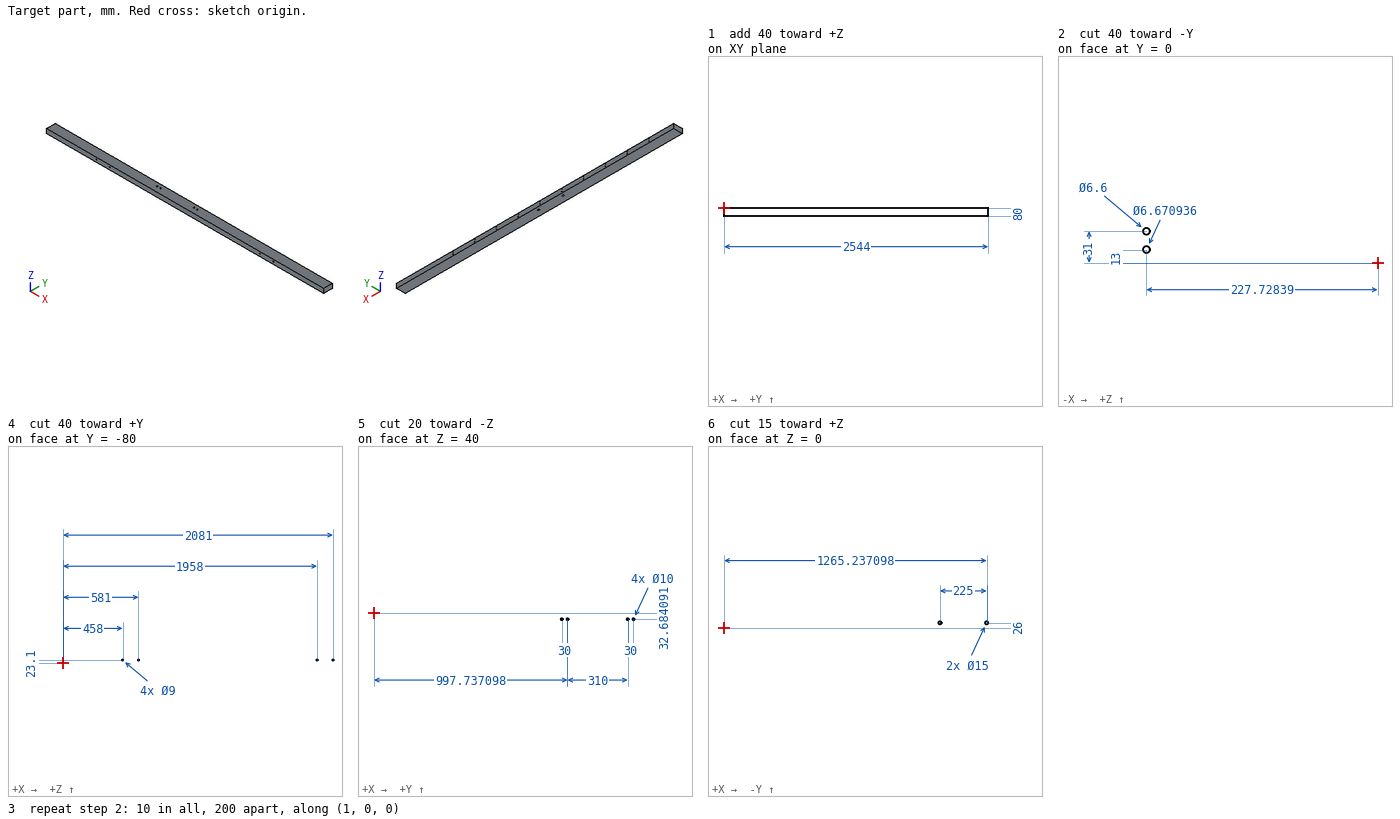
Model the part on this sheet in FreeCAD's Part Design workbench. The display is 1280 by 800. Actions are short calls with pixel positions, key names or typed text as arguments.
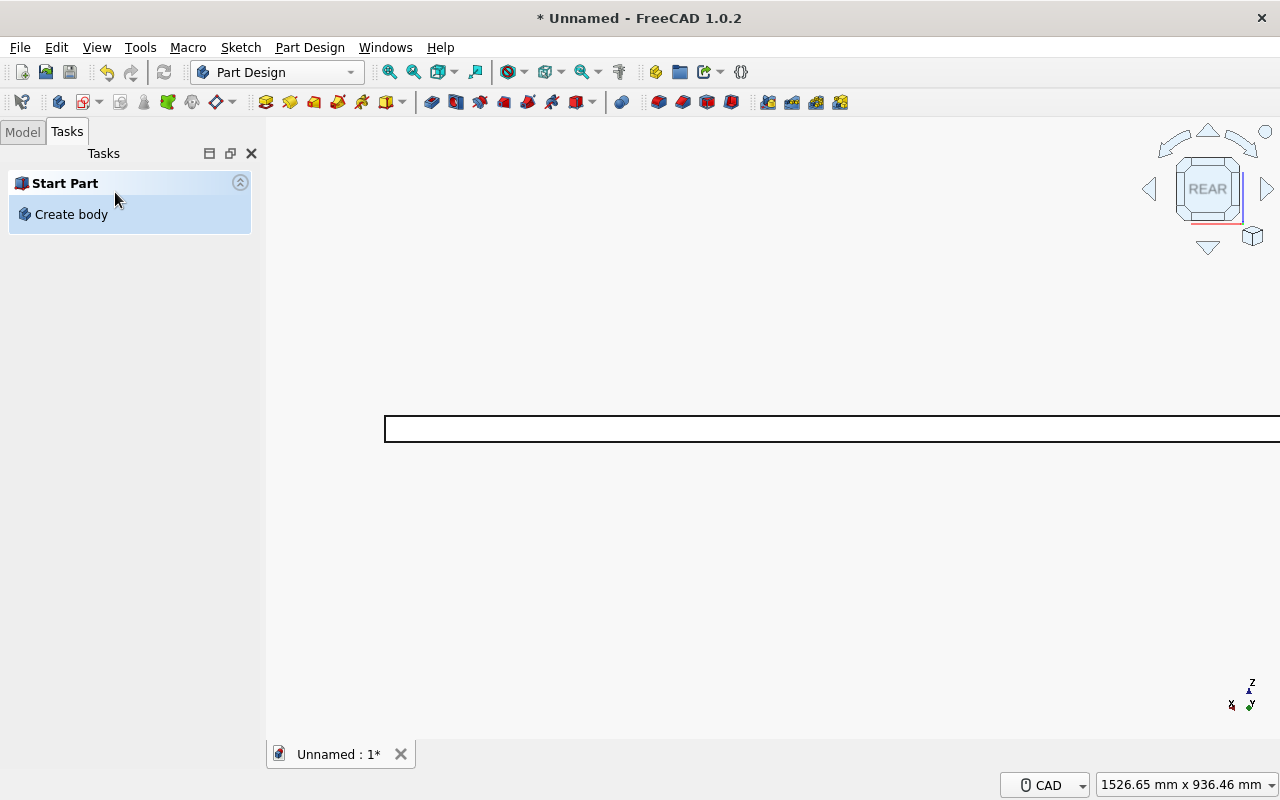
key(v)
key(f)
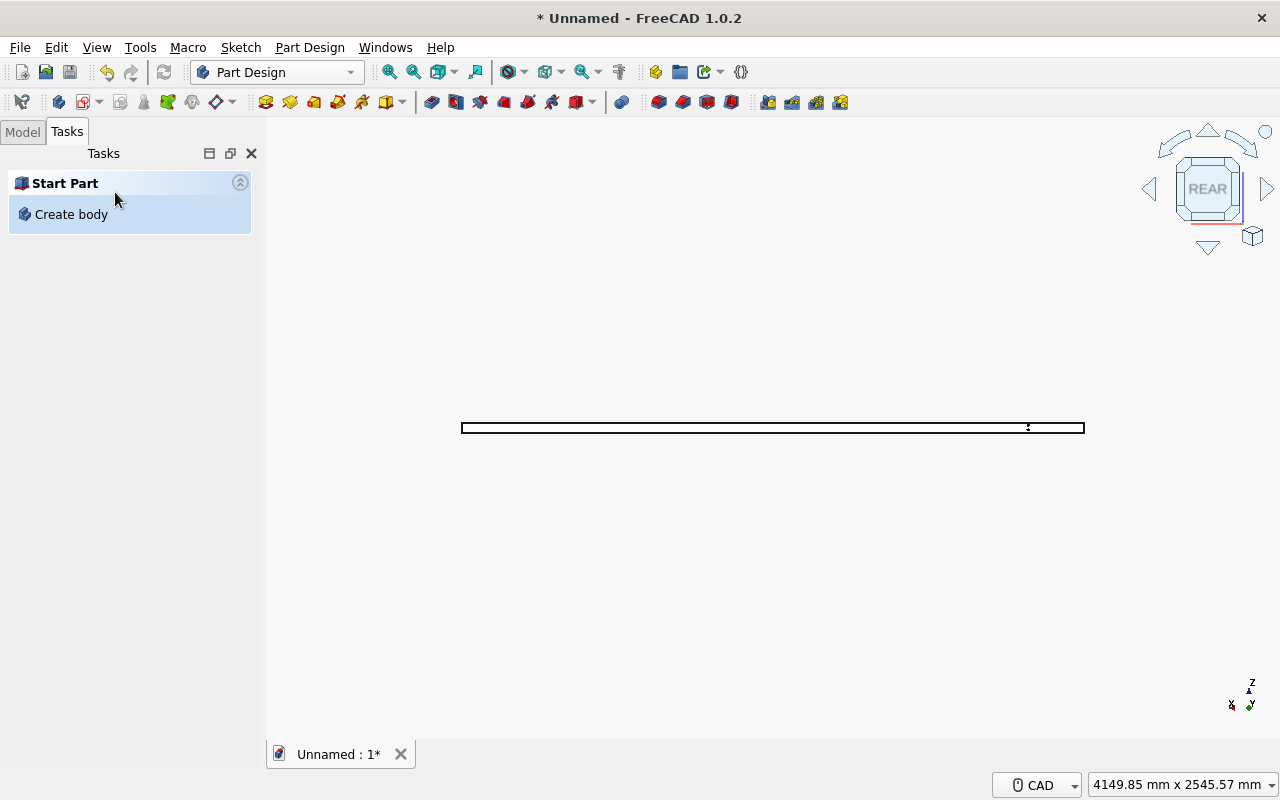
click(23, 131)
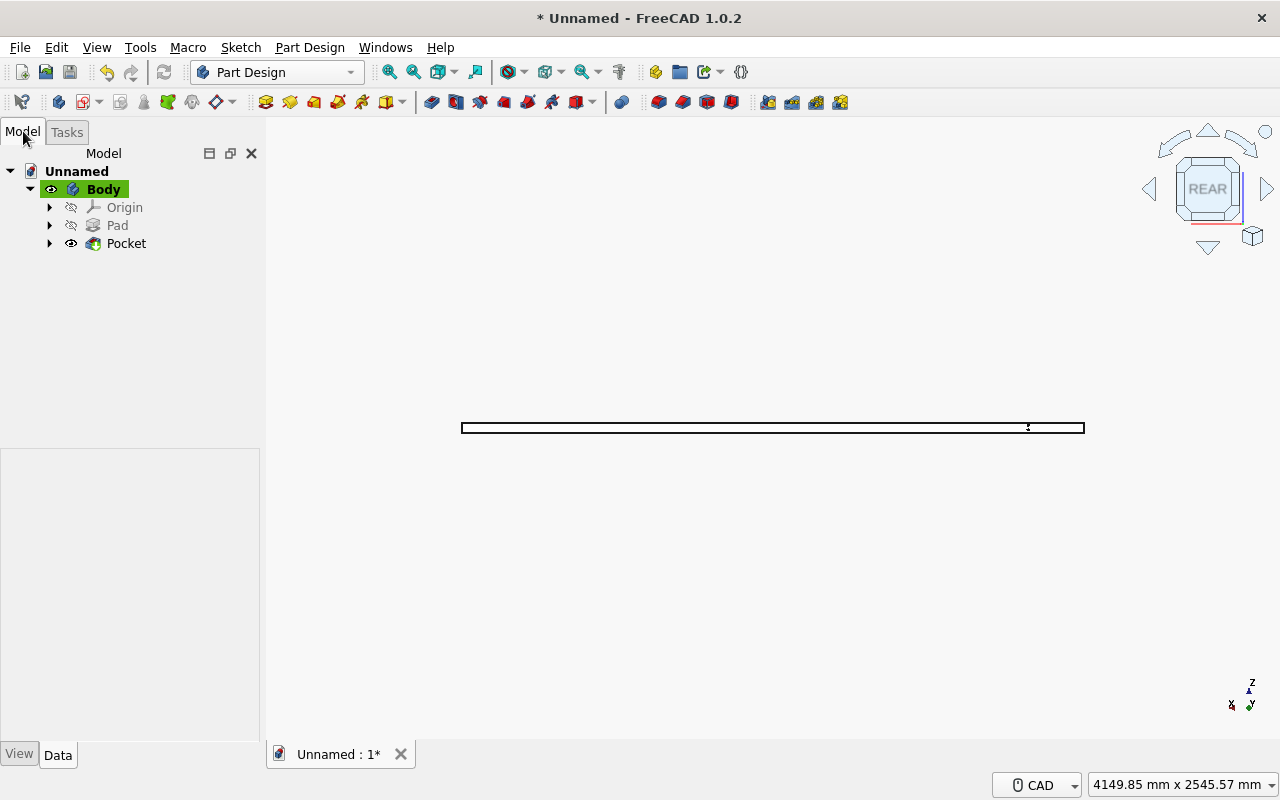
click(116, 243)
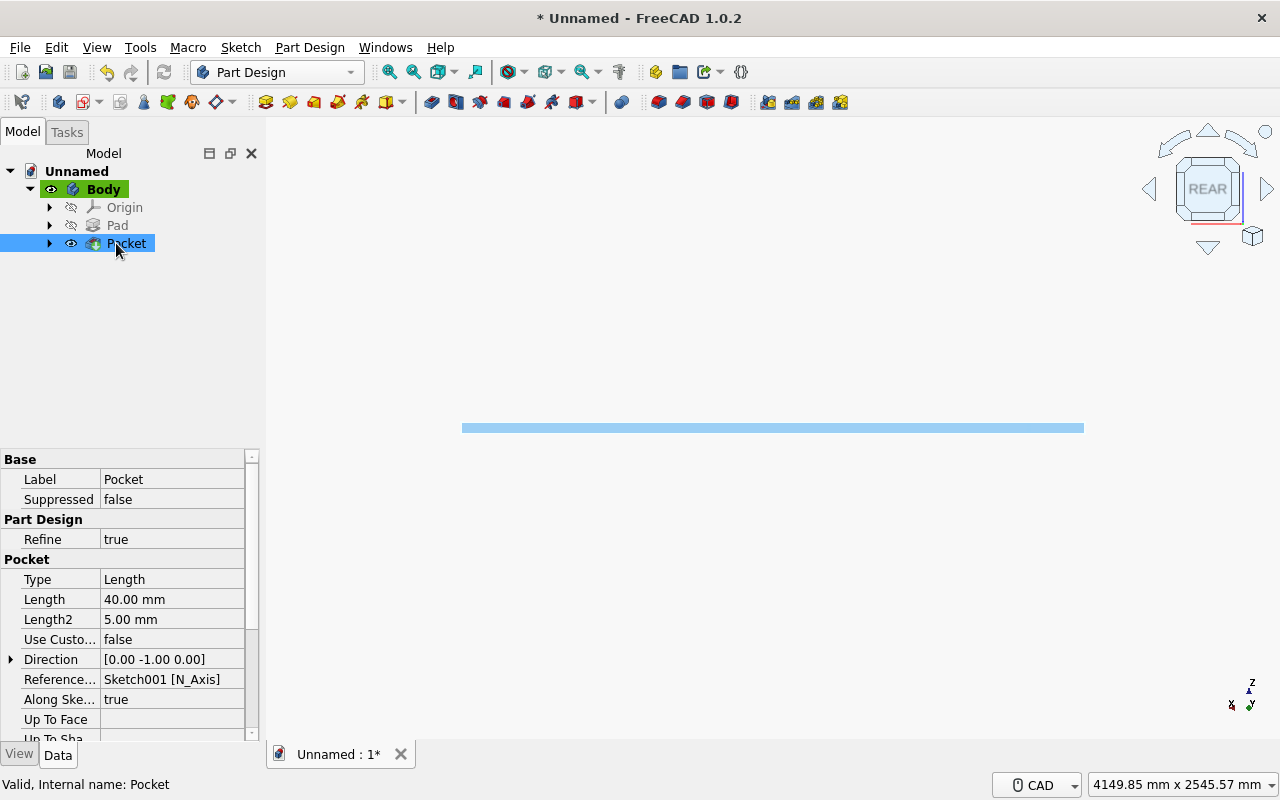
click(792, 102)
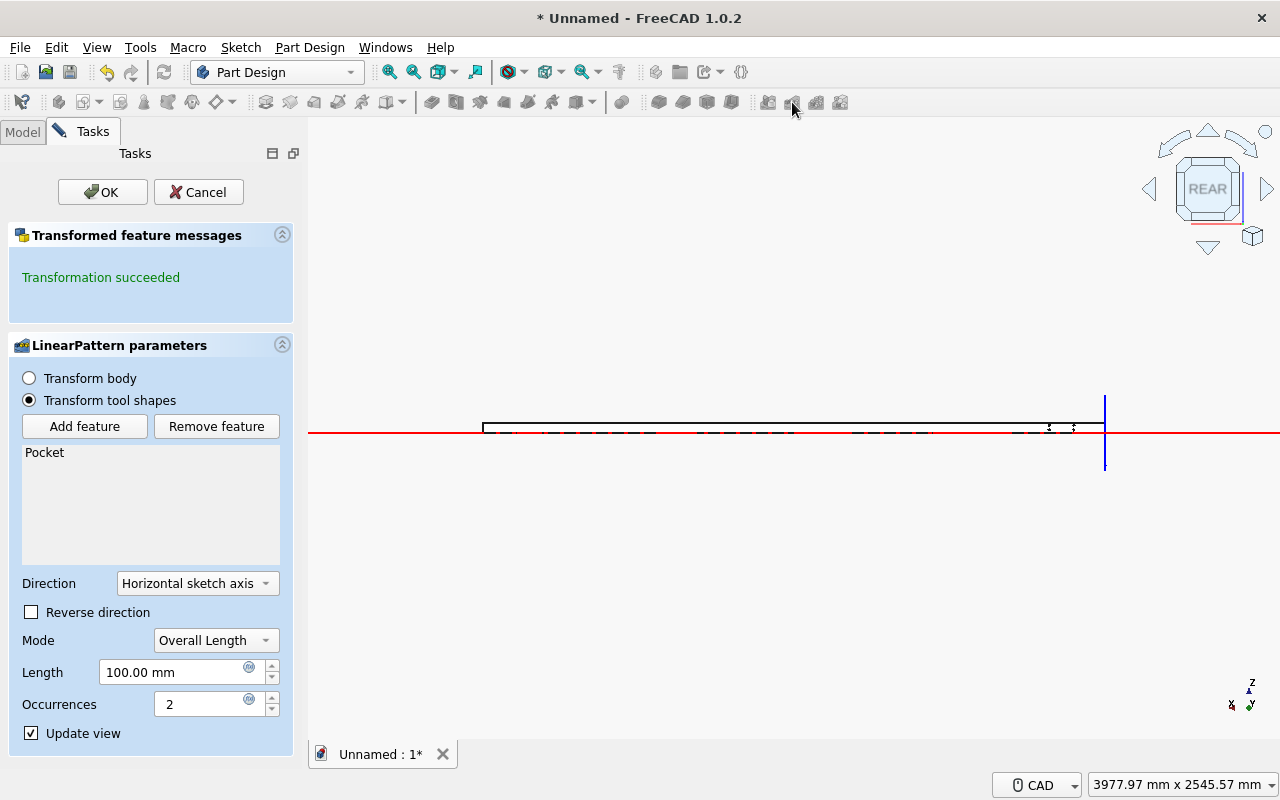
click(198, 584)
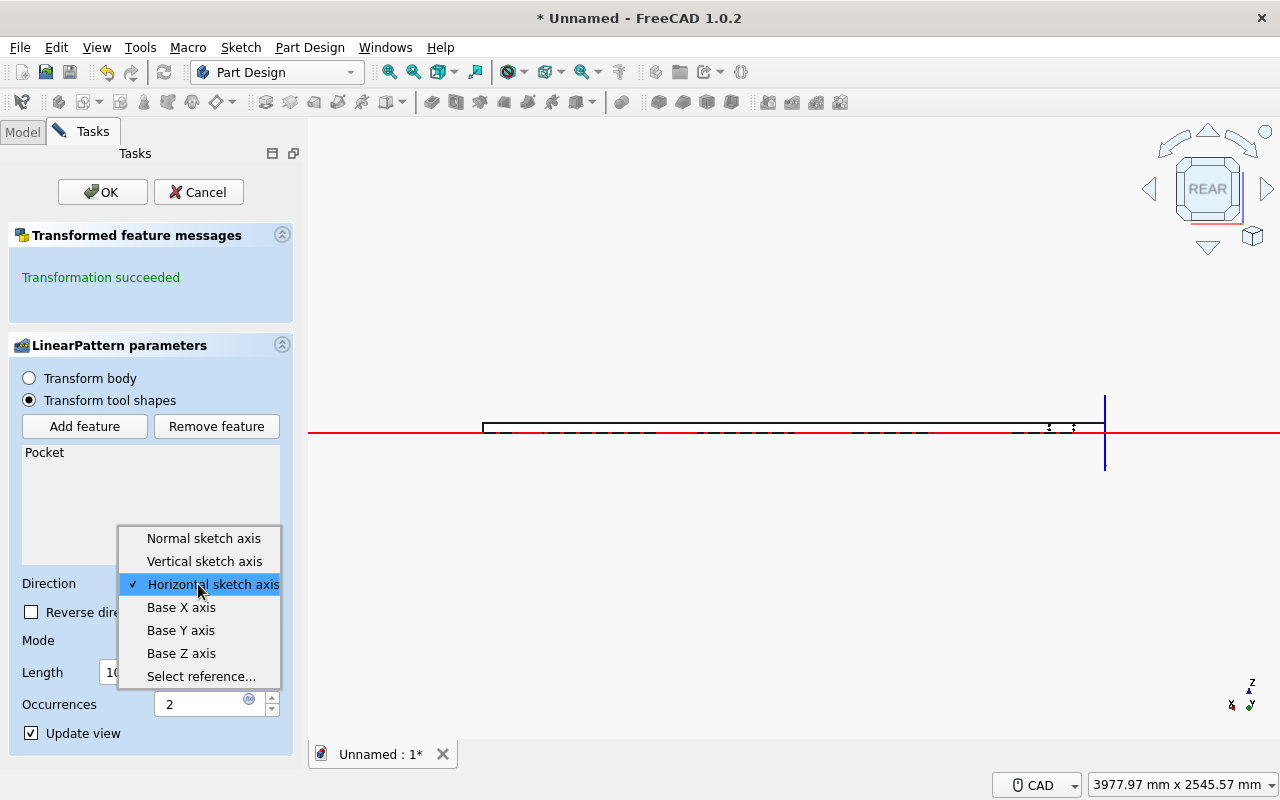
click(198, 608)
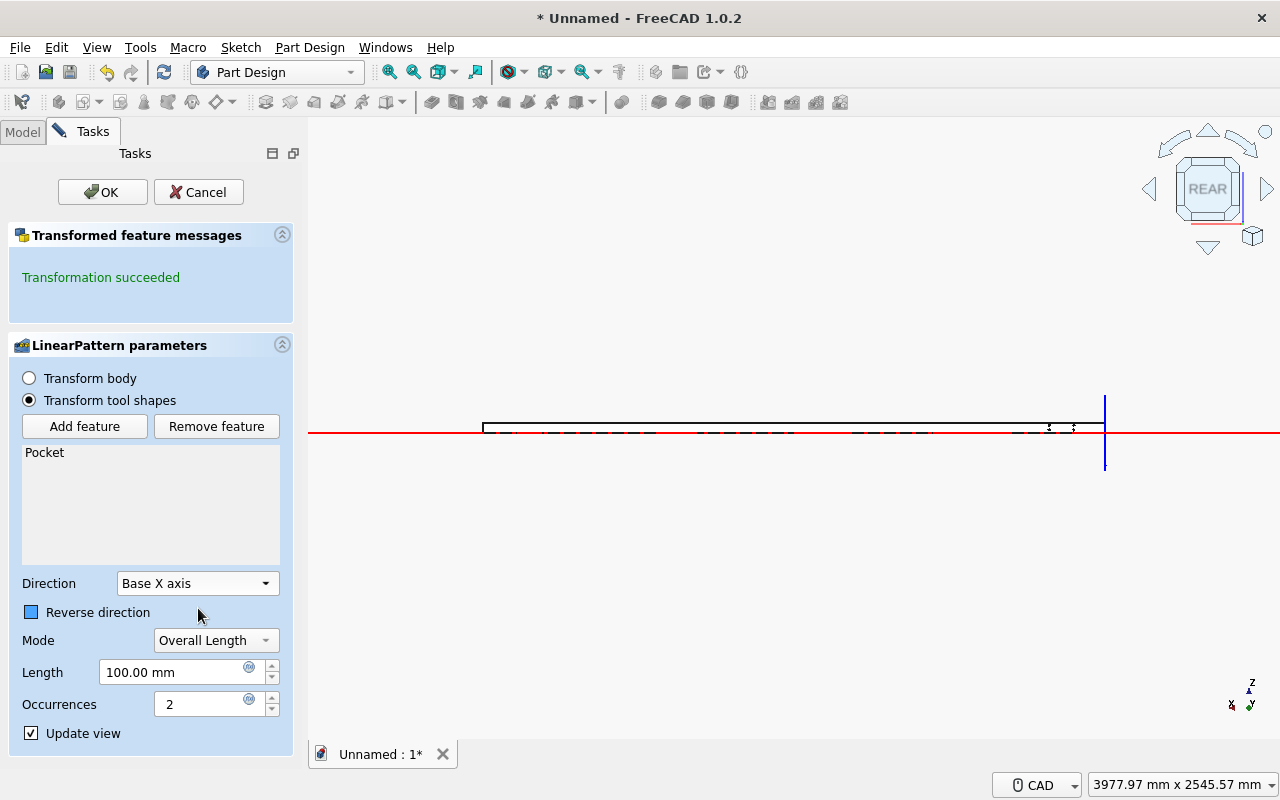
click(217, 640)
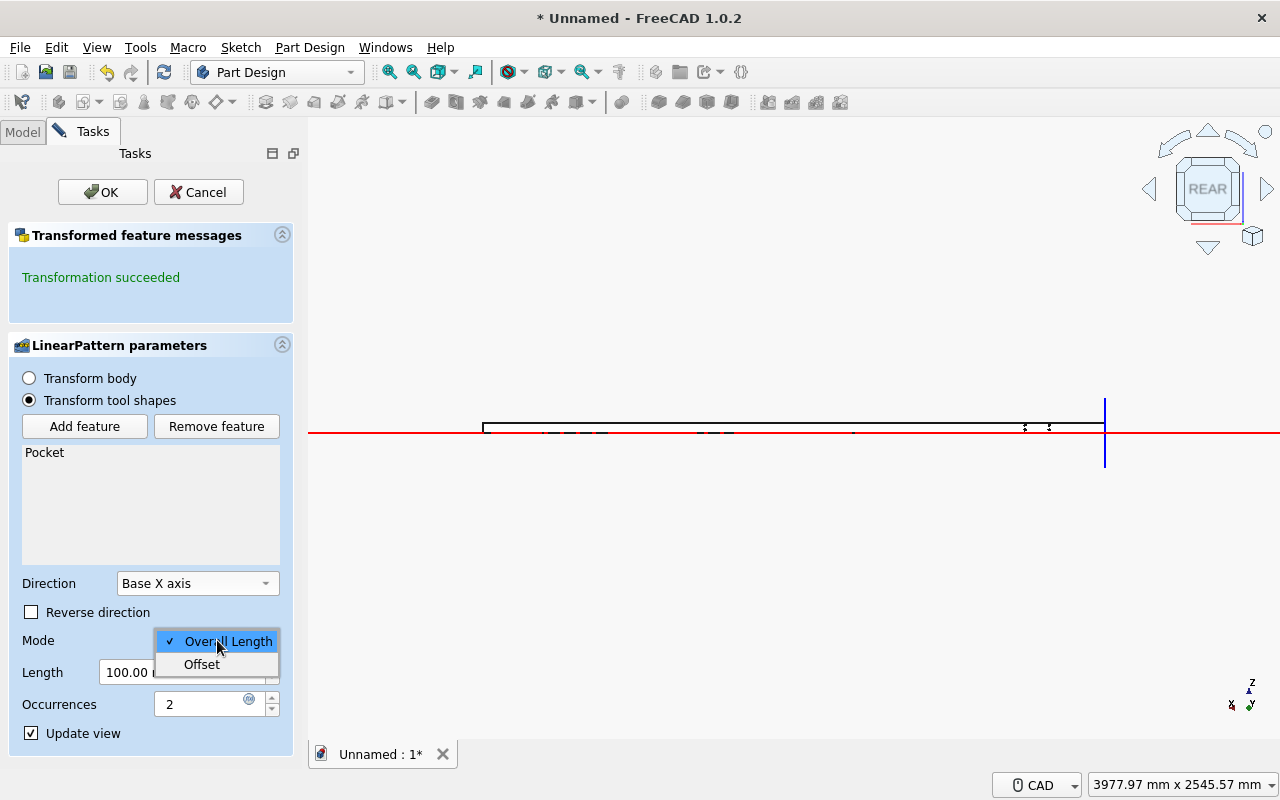
click(216, 664)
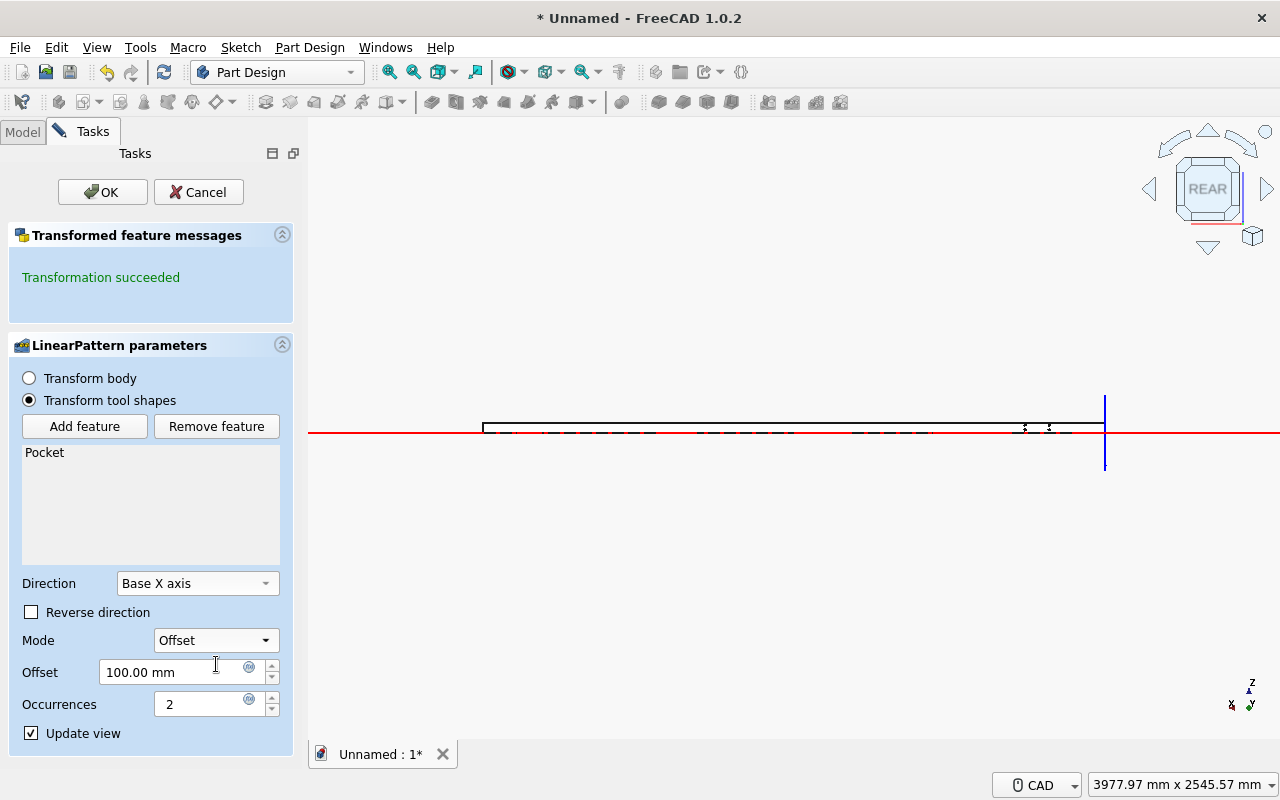
triple_click(182, 672)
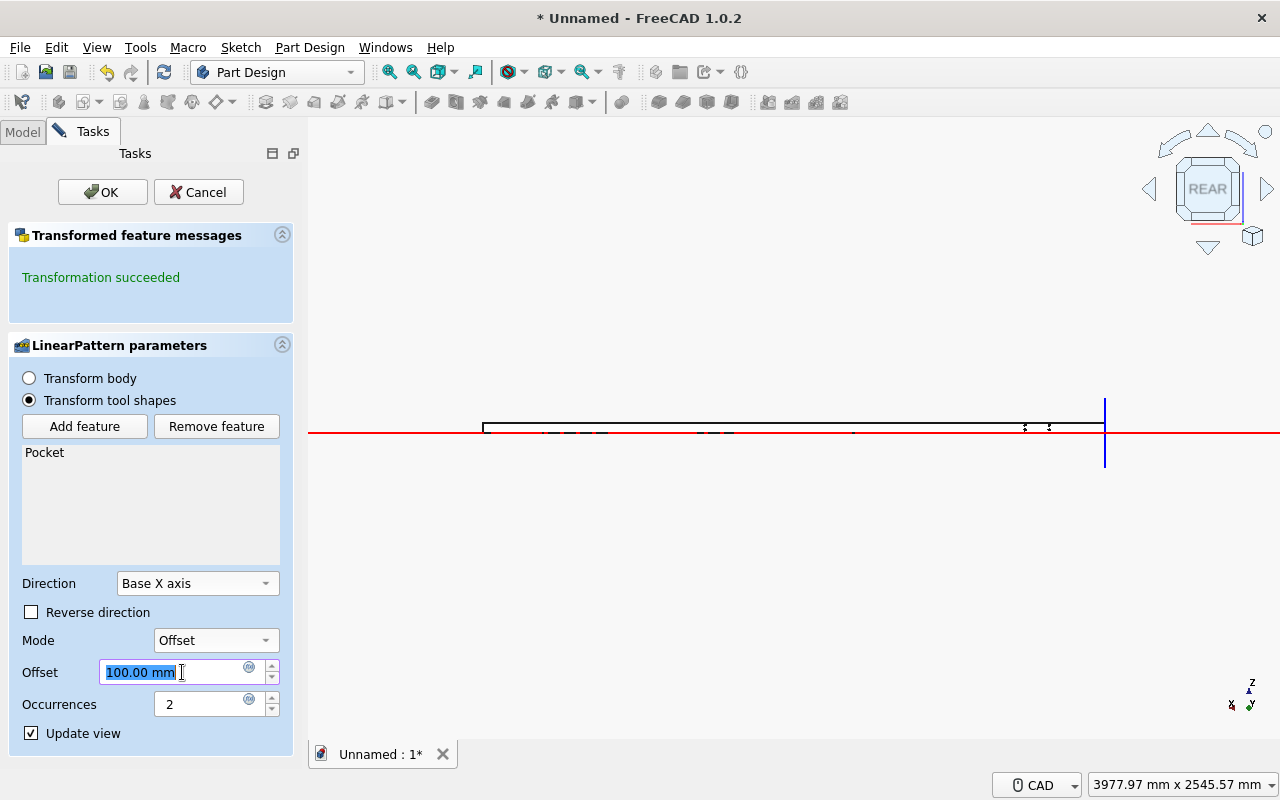
text(200)
key(Tab)